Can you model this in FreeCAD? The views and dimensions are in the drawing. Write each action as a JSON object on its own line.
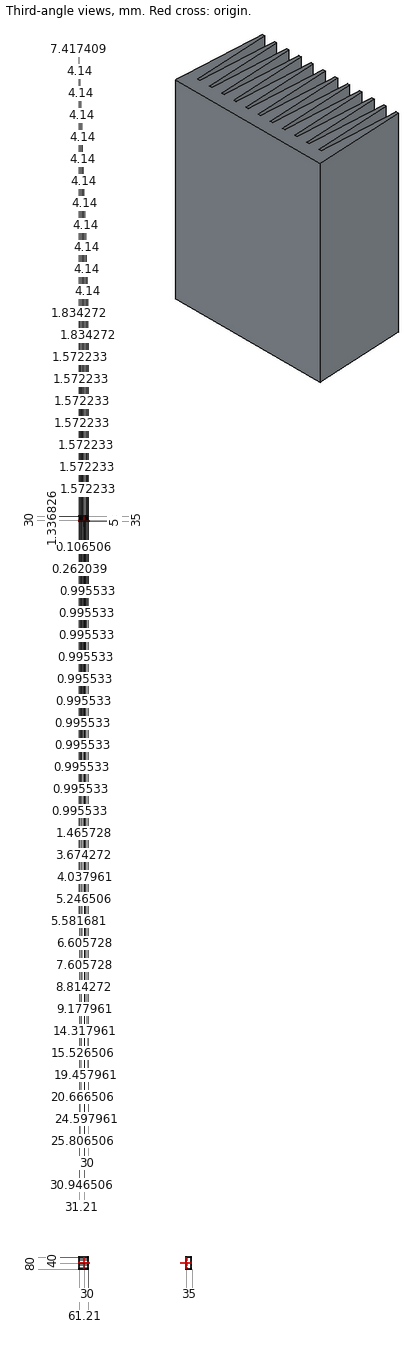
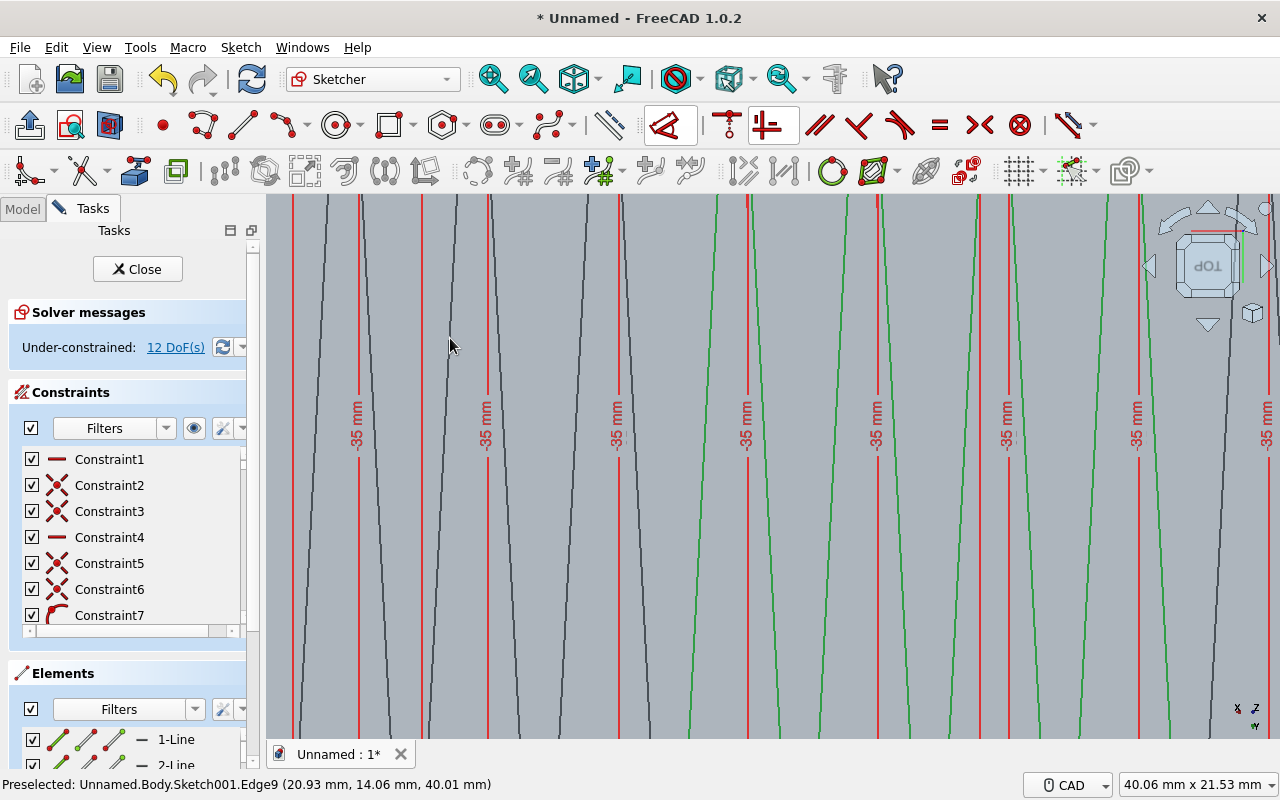
{"action": "left_click", "coordinate": [580, 338]}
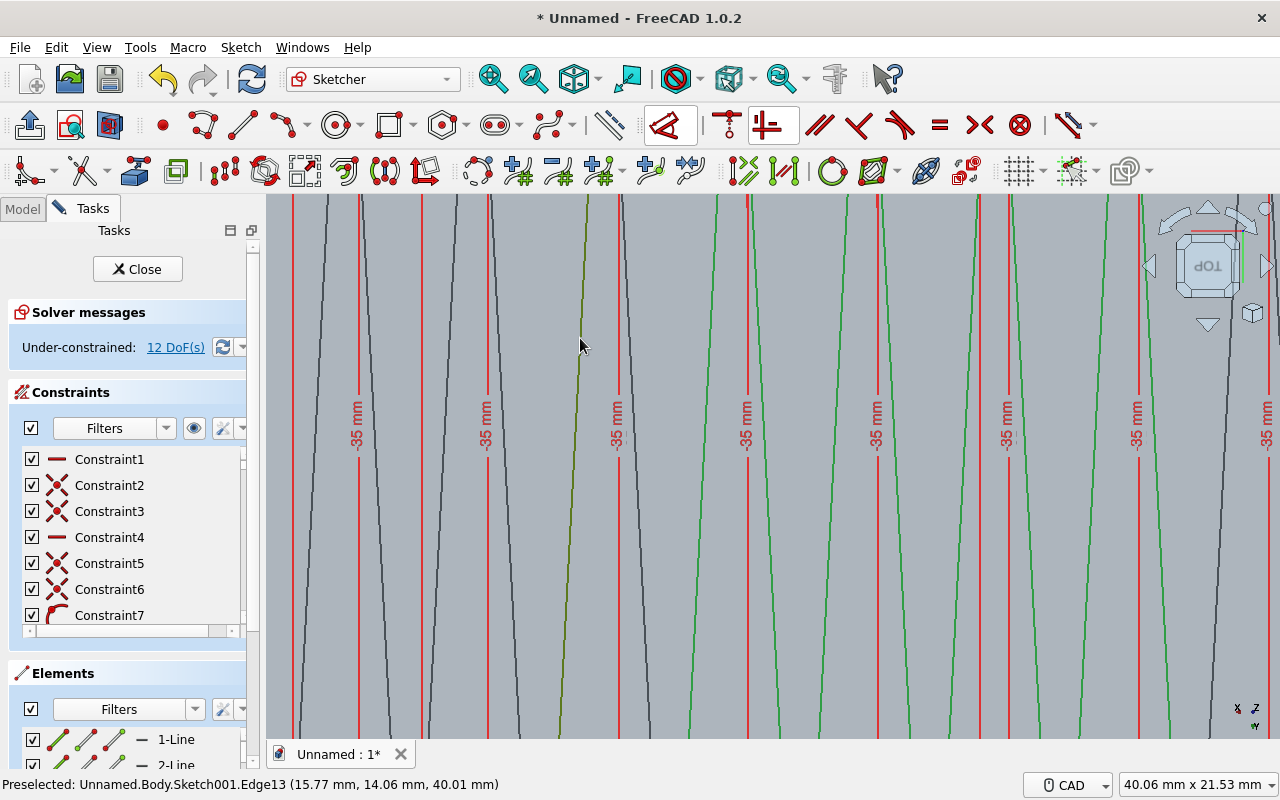
{"action": "key", "text": "l"}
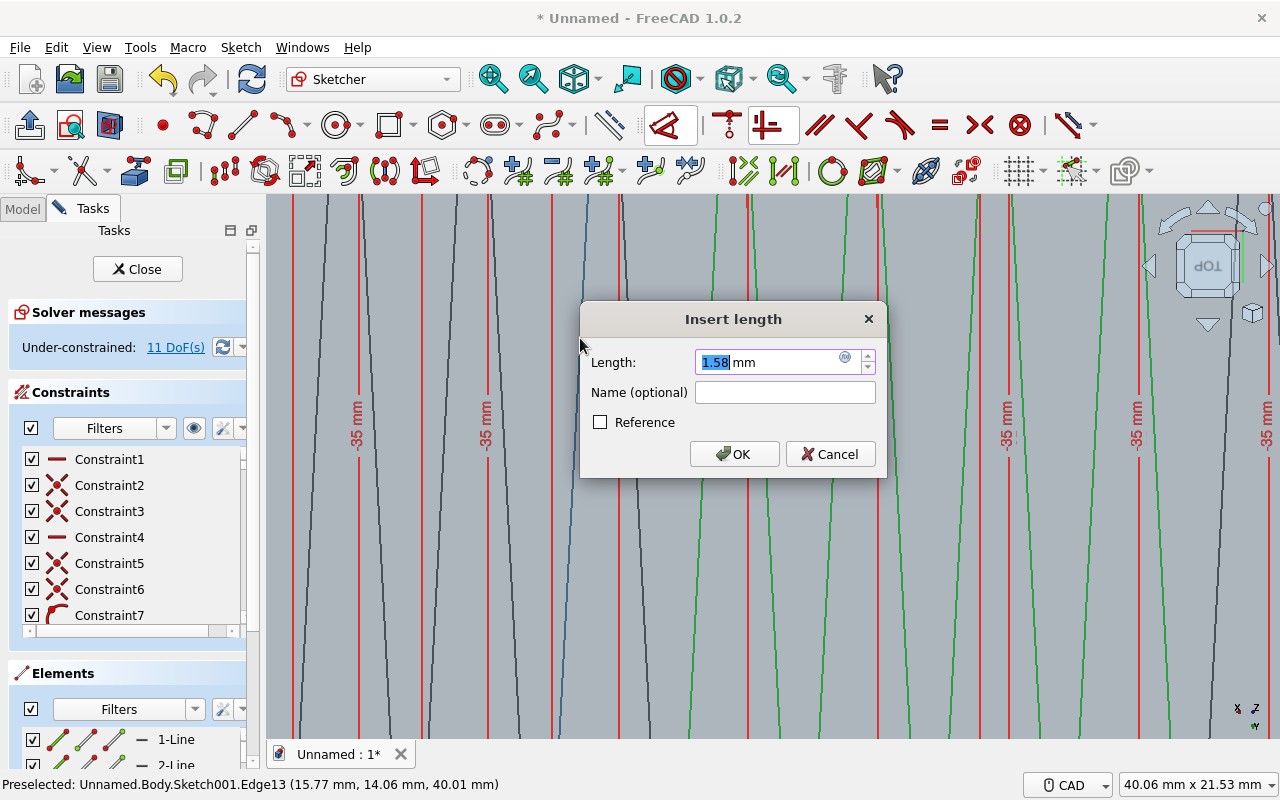
{"action": "type", "text": "1.572233"}
{"action": "key", "text": "Return"}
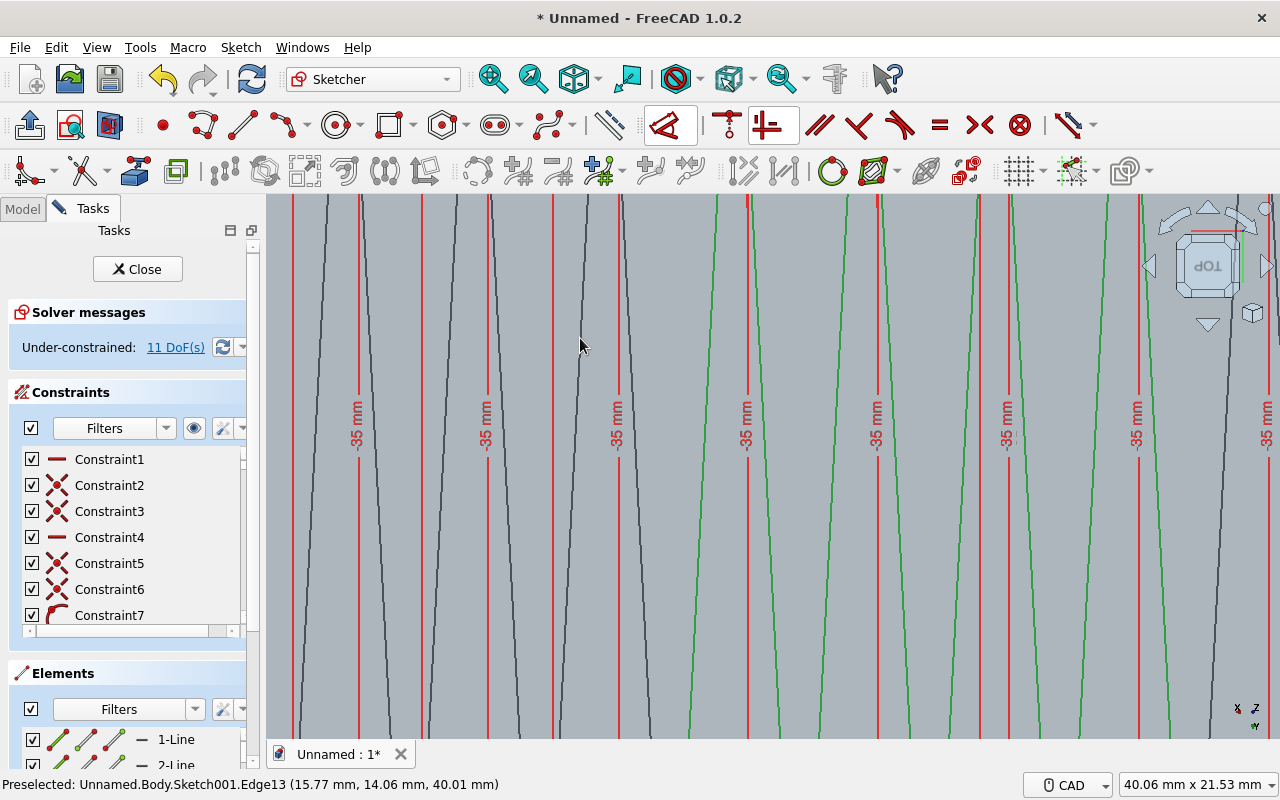
{"action": "scroll", "coordinate": [536, 490], "scroll_direction": "down", "scroll_amount": 5}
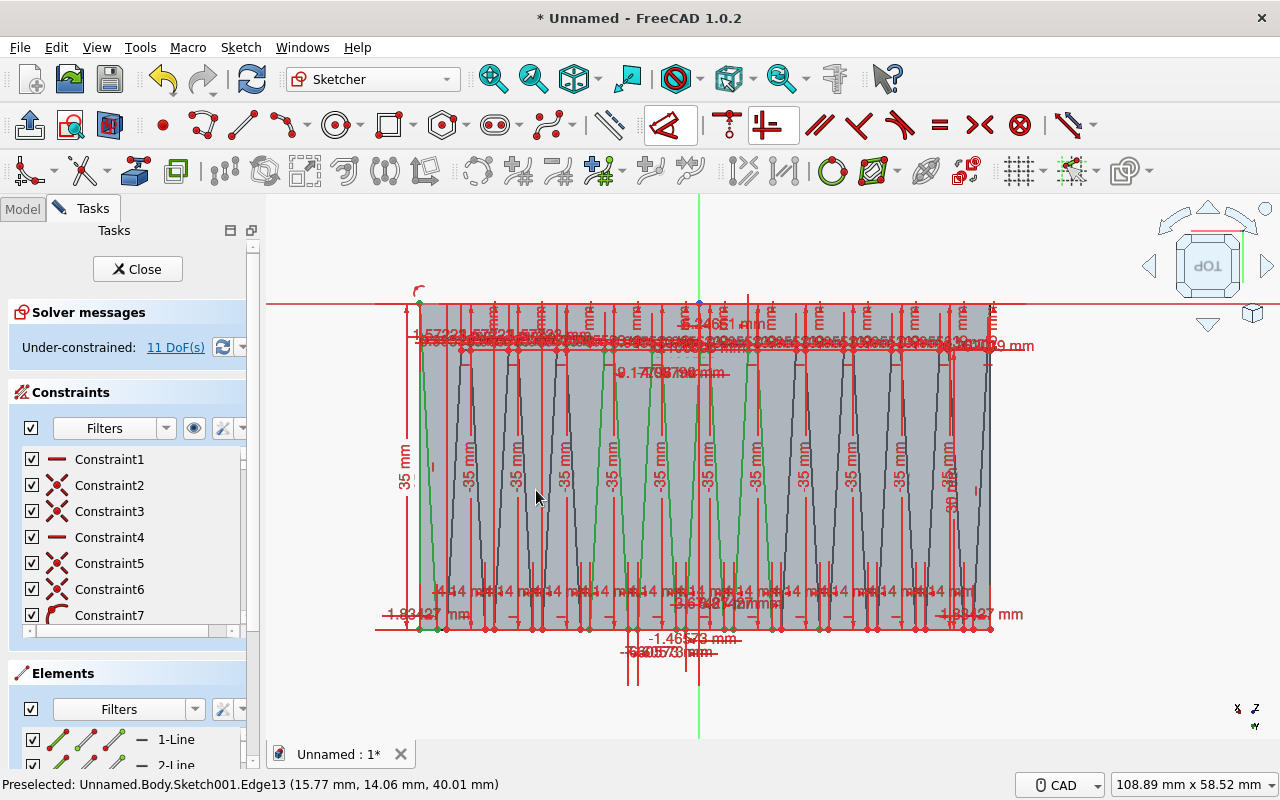
{"action": "scroll", "coordinate": [792, 434], "scroll_direction": "up", "scroll_amount": 5}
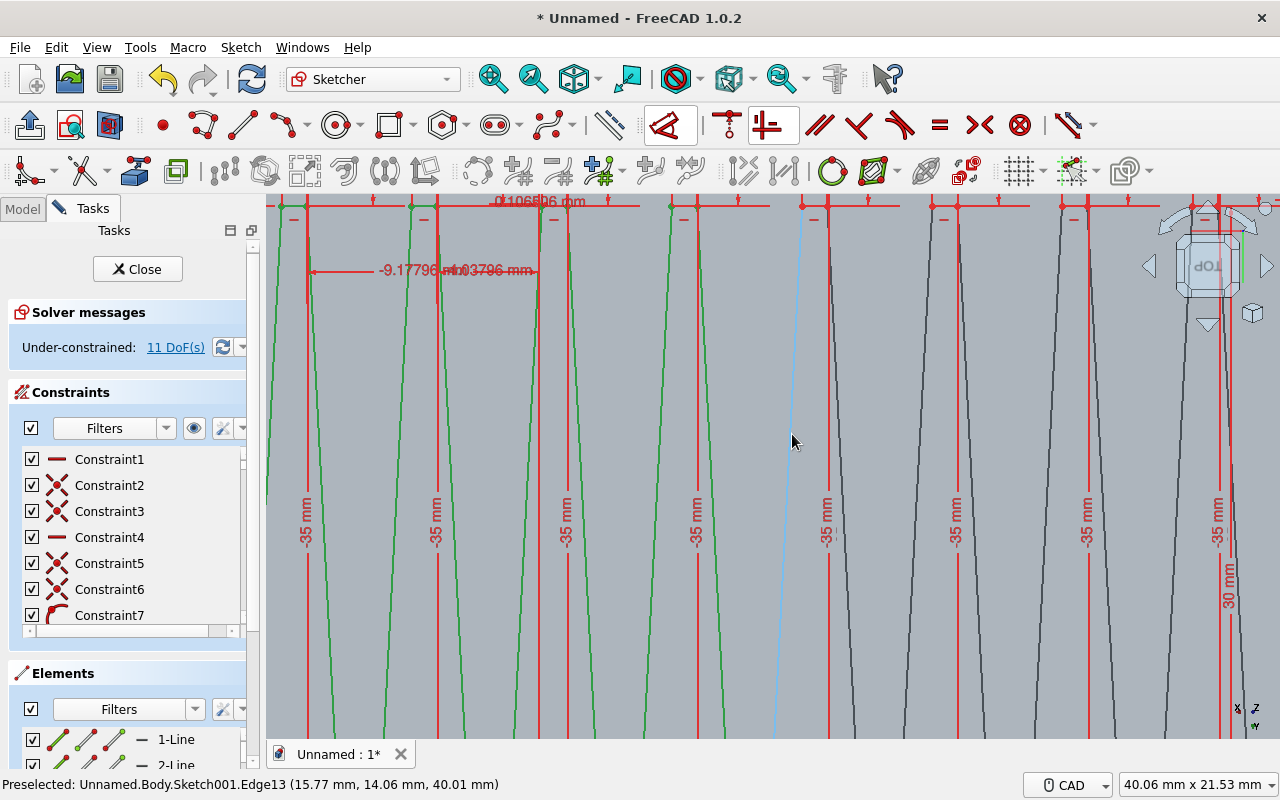
{"action": "left_click", "coordinate": [790, 434]}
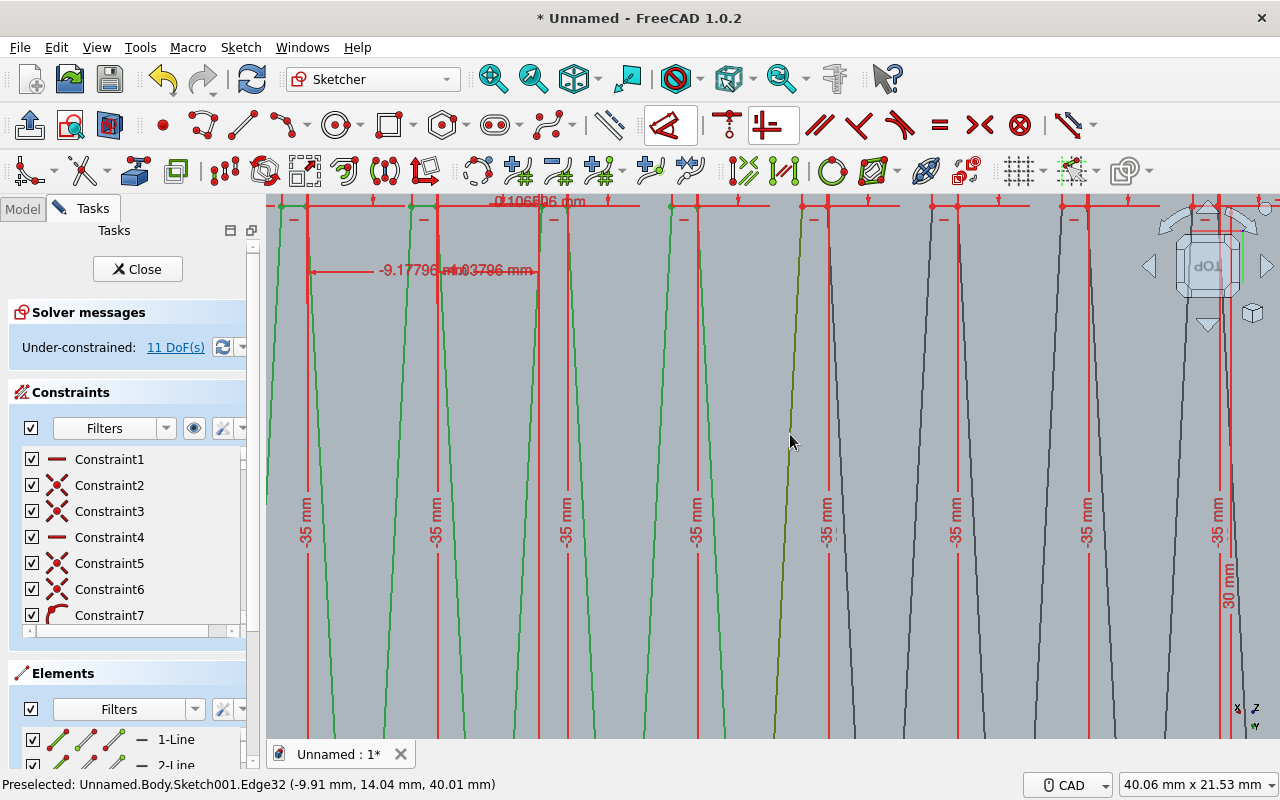
{"action": "left_click", "coordinate": [692, 126]}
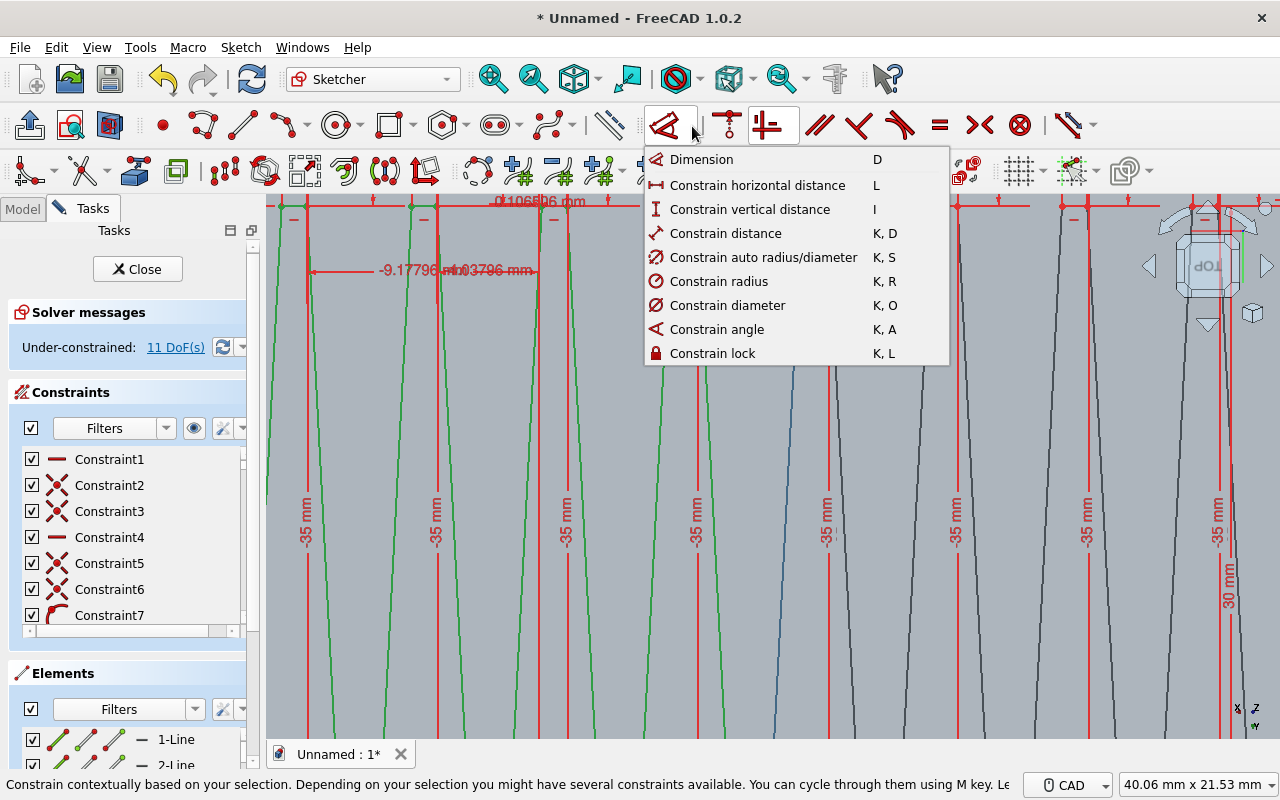
{"action": "left_click", "coordinate": [797, 185]}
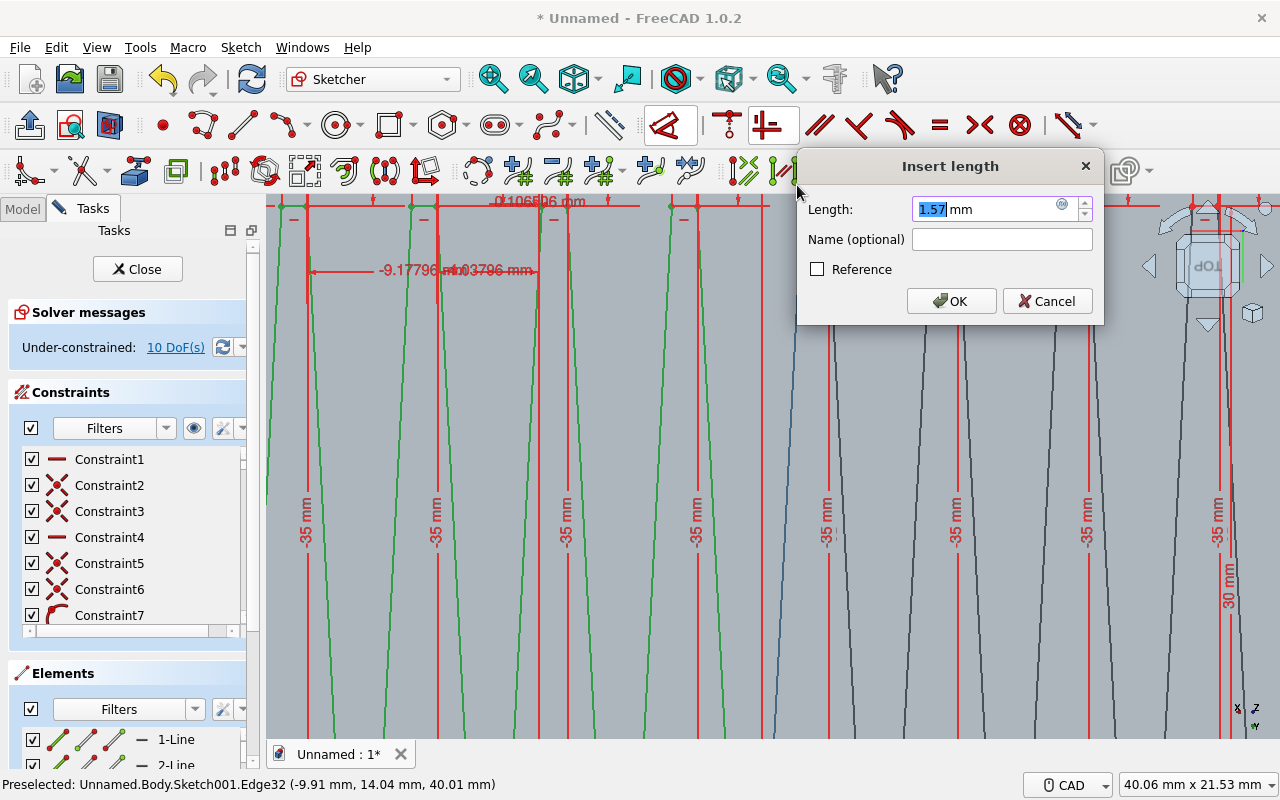
{"action": "type", "text": "1.572233"}
{"action": "key", "text": "Return"}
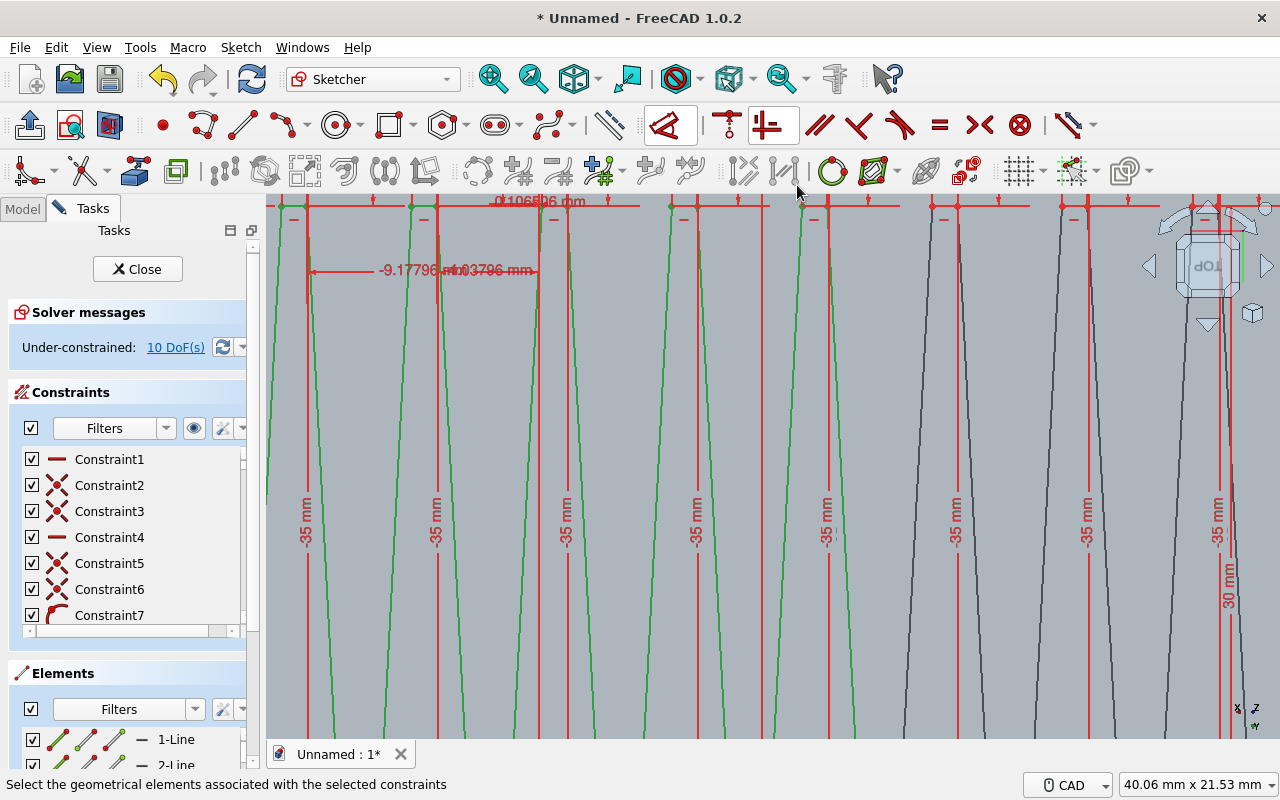
{"action": "left_click", "coordinate": [920, 434]}